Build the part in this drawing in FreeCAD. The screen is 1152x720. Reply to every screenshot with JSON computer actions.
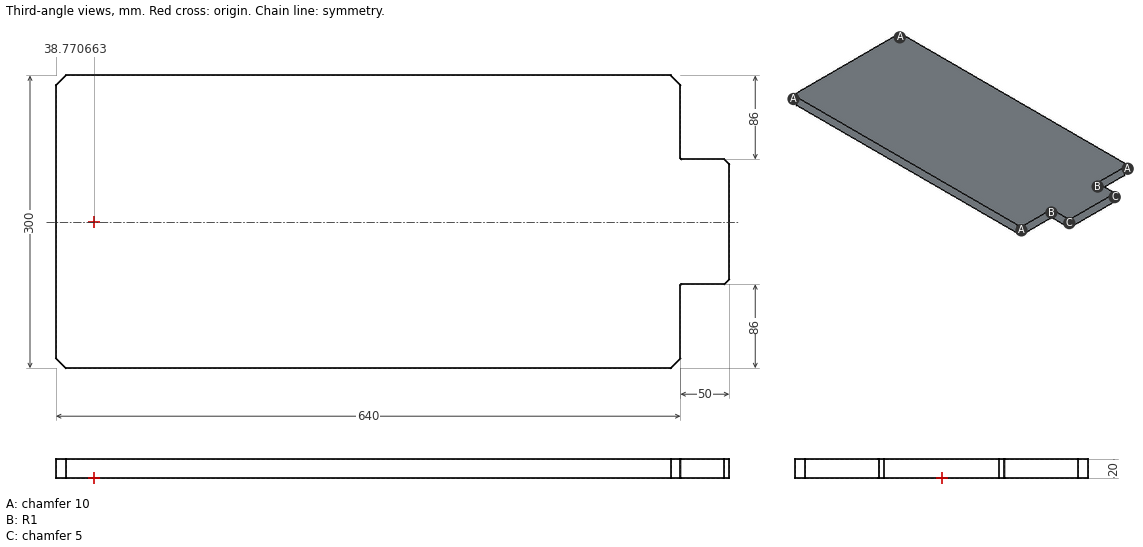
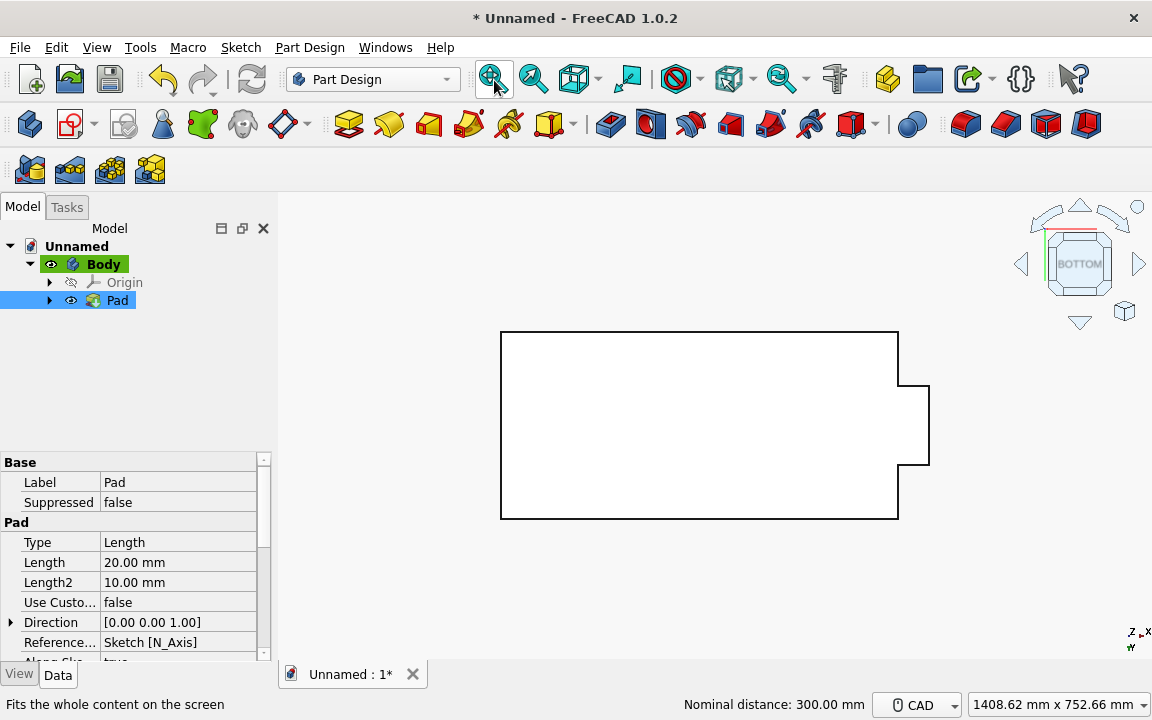
{"action": "scroll", "coordinate": [501, 331], "scroll_direction": "up", "scroll_amount": 6}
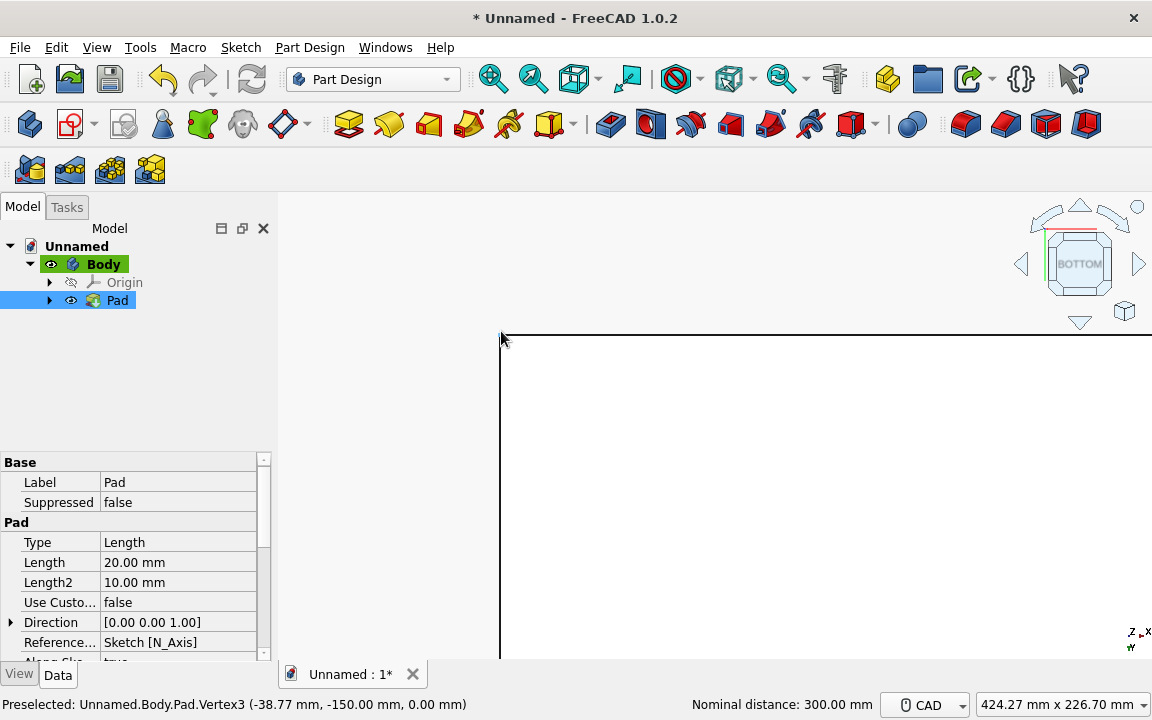
{"action": "left_click", "coordinate": [494, 80]}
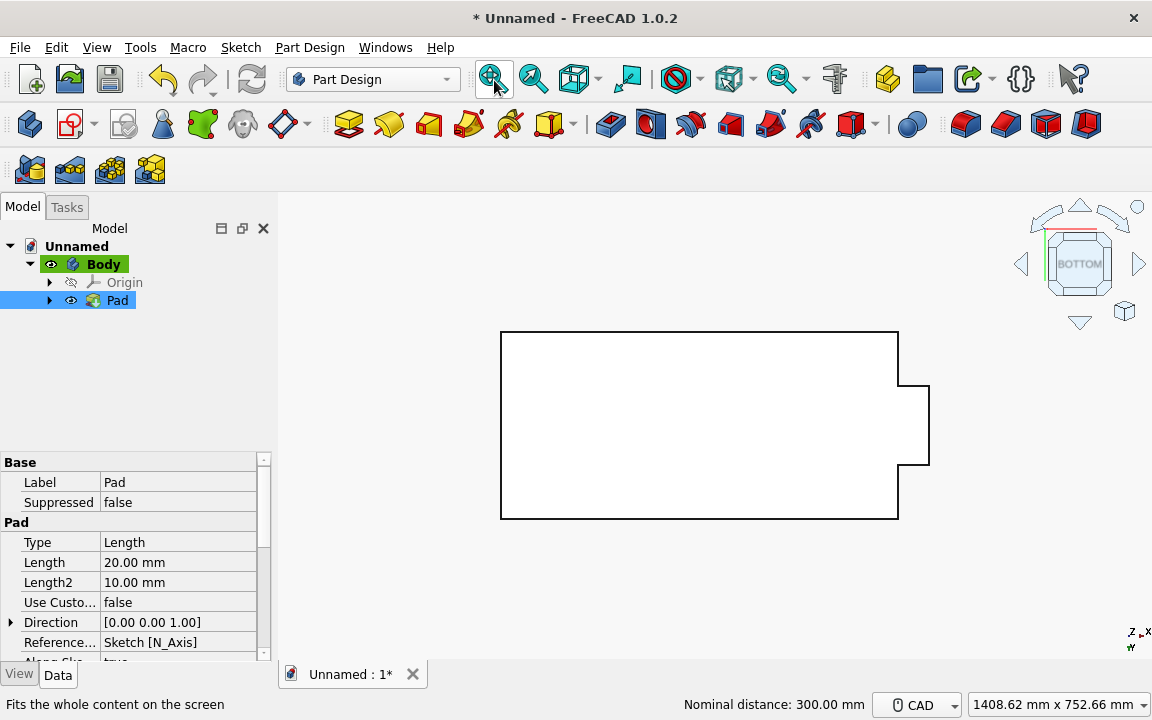
{"action": "key", "text": "4"}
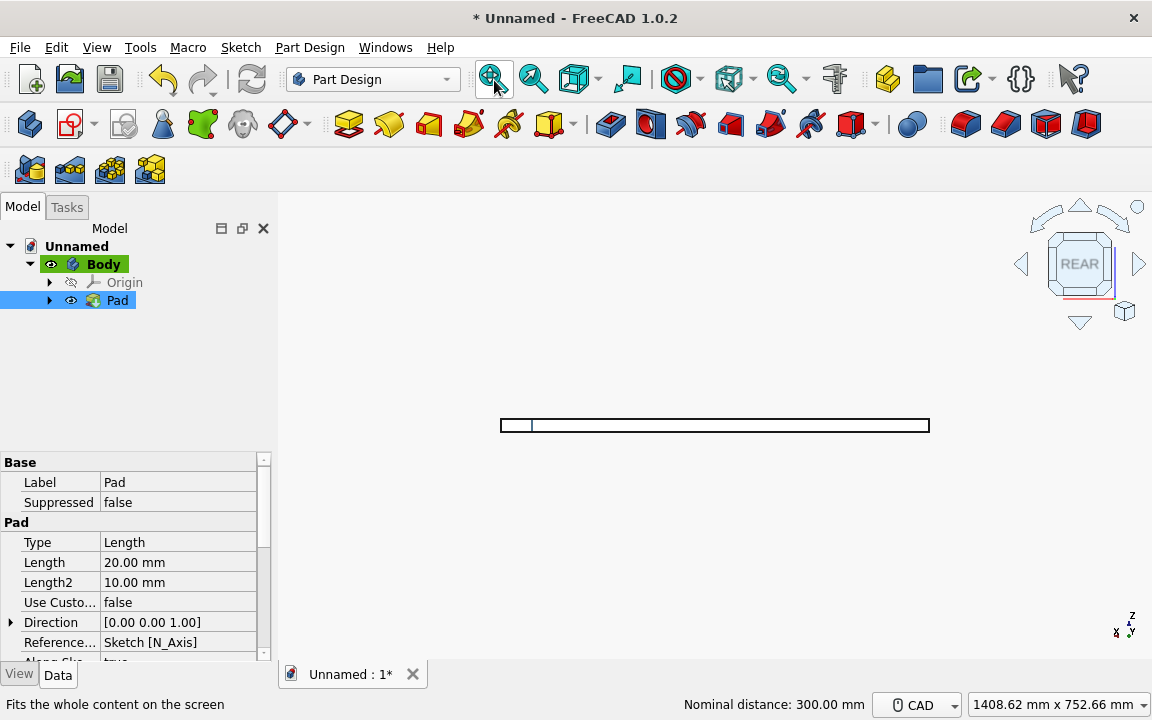
{"action": "scroll", "coordinate": [929, 424], "scroll_direction": "up", "scroll_amount": 6}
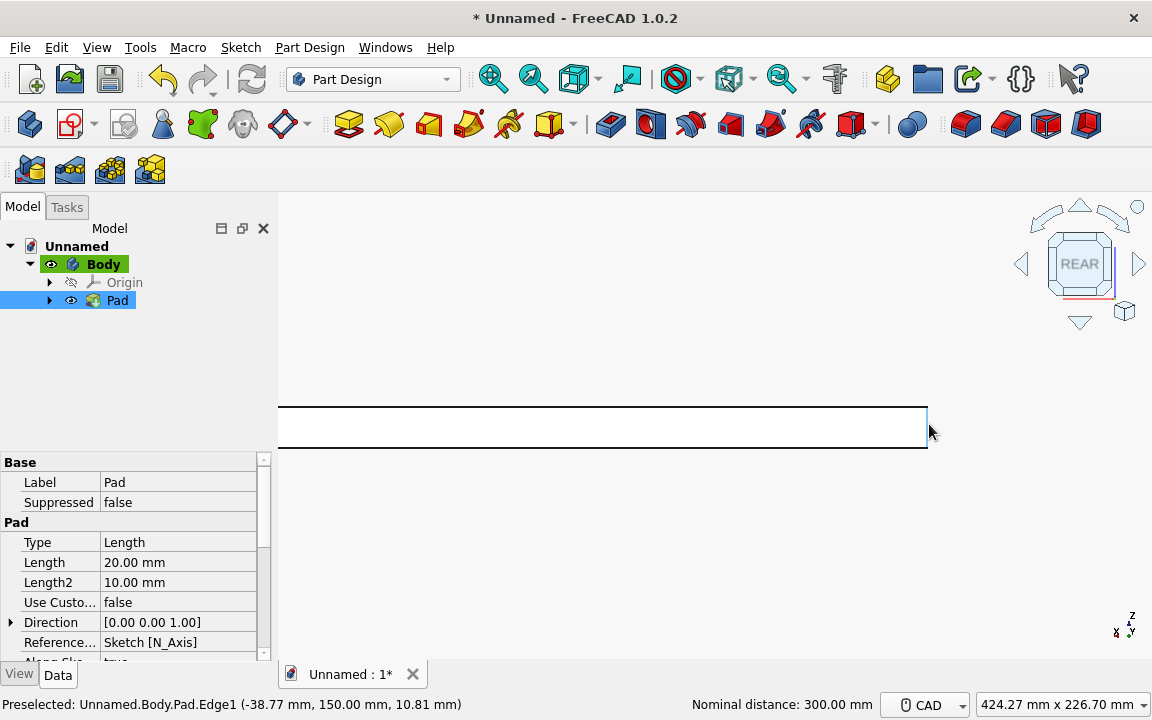
{"action": "left_click", "coordinate": [927, 427], "text": "ctrl"}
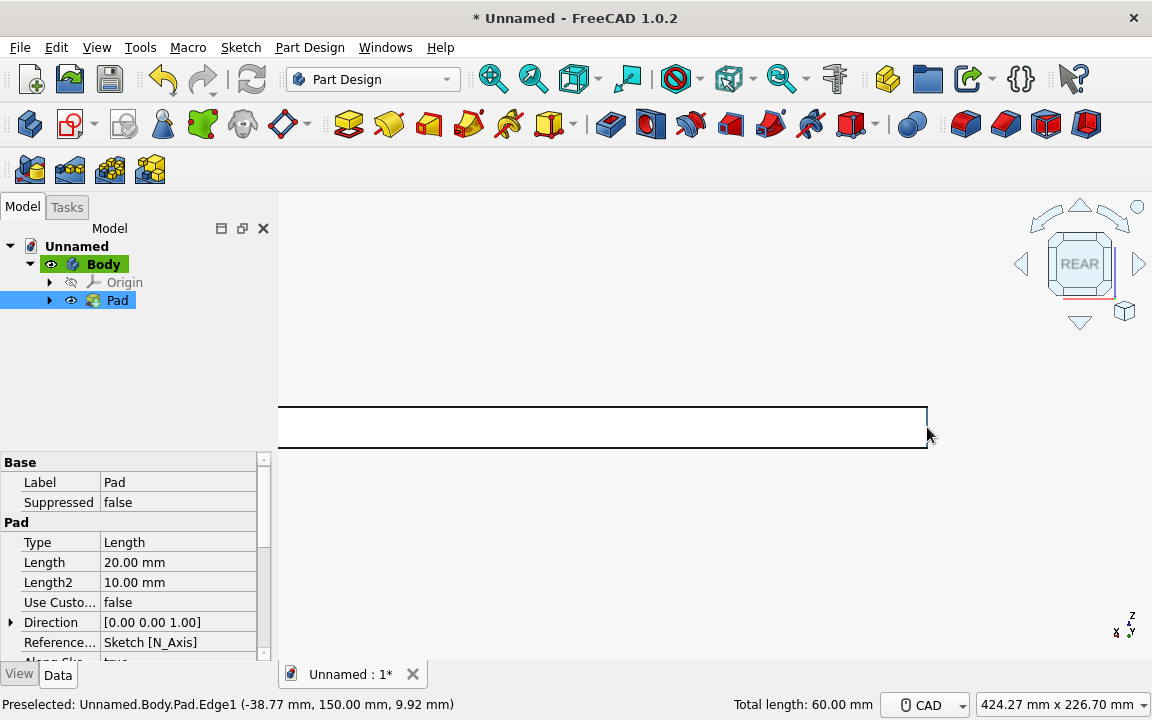
{"action": "left_click", "coordinate": [494, 80]}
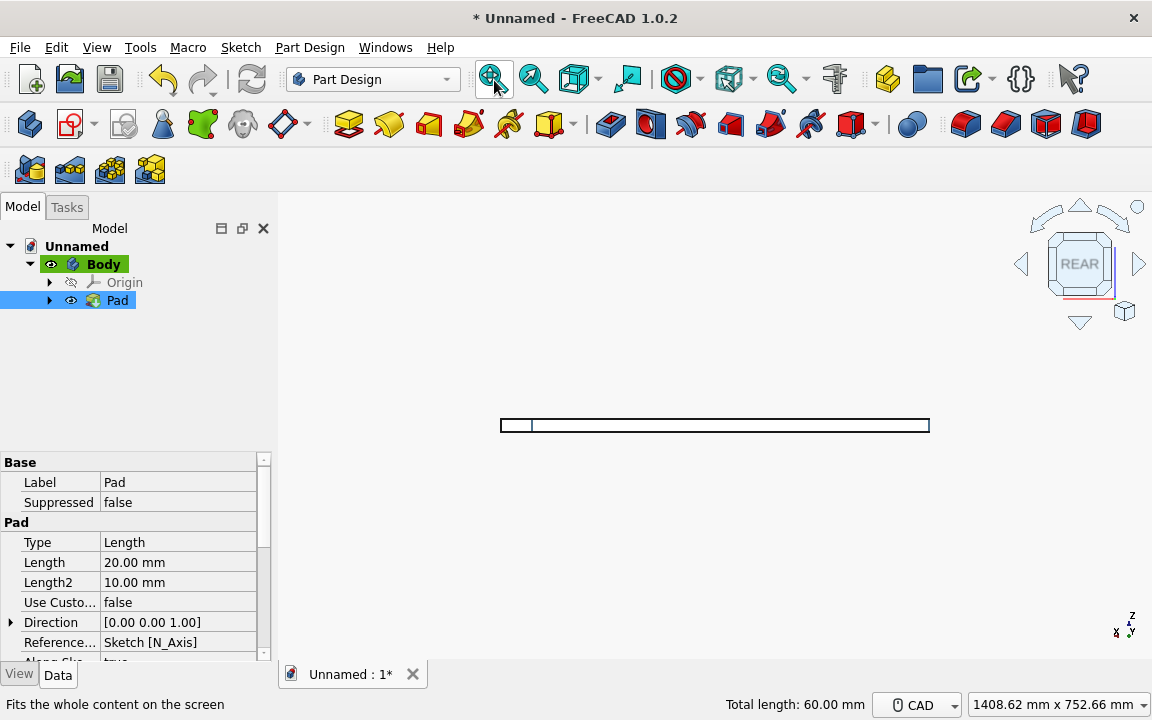
{"action": "key", "text": "6"}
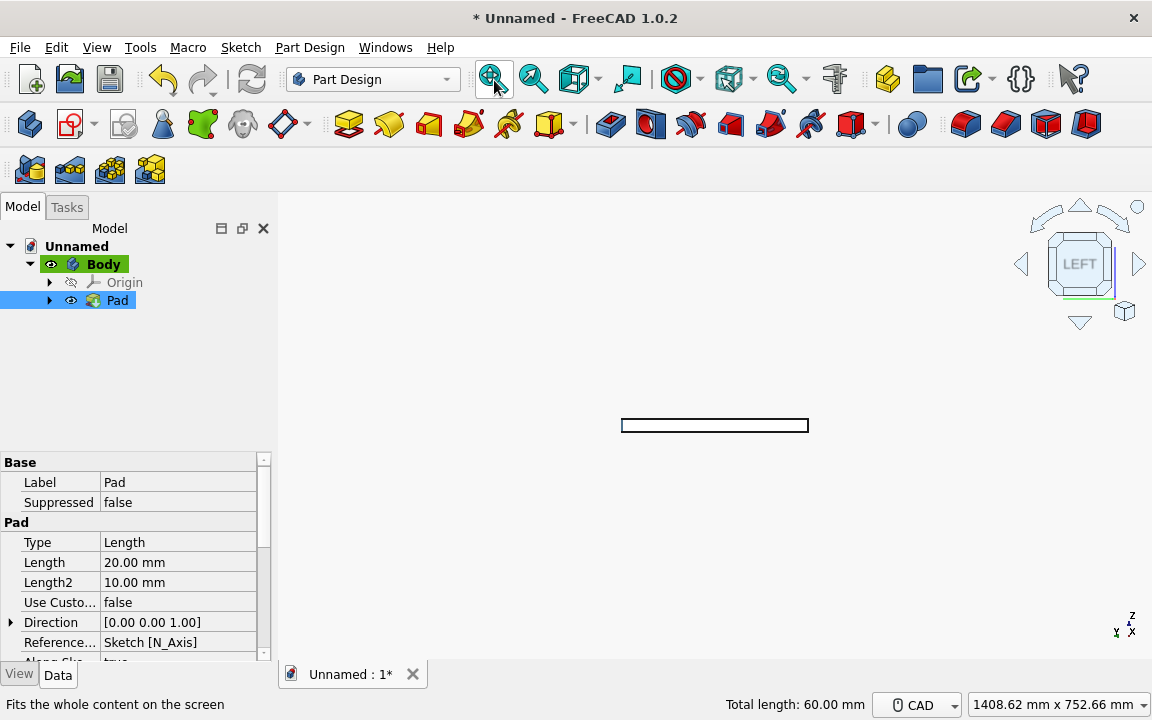
{"action": "left_click", "coordinate": [494, 80]}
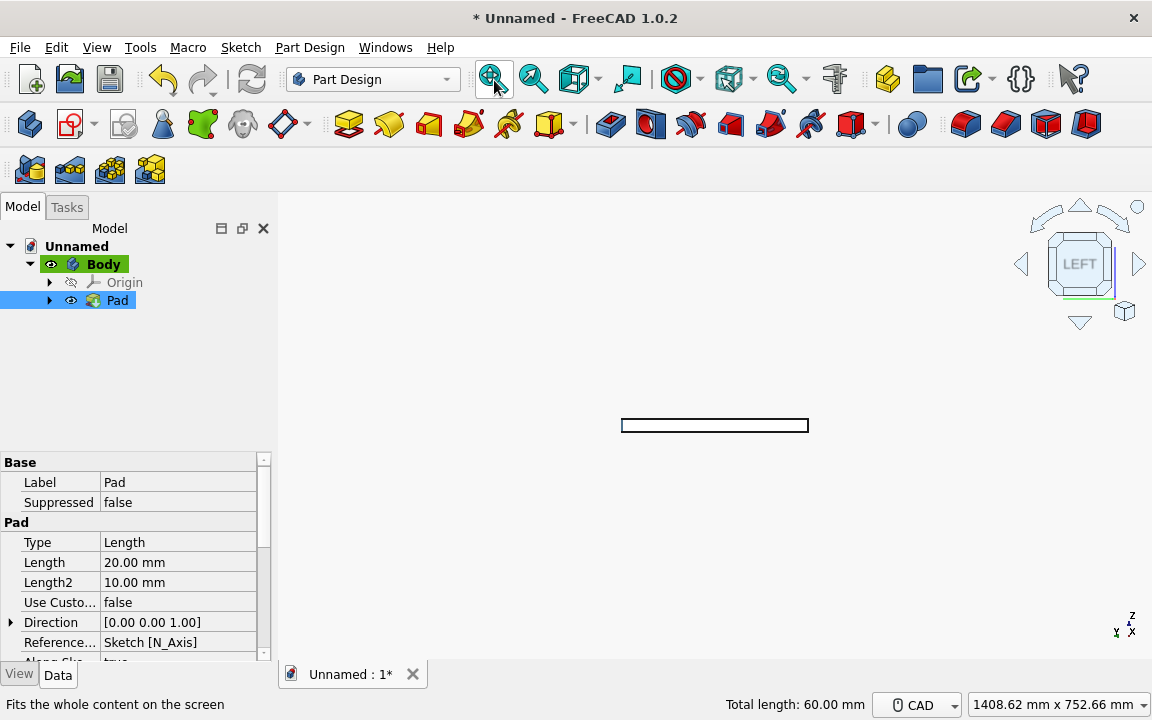
{"action": "scroll", "coordinate": [808, 424], "scroll_direction": "up", "scroll_amount": 6}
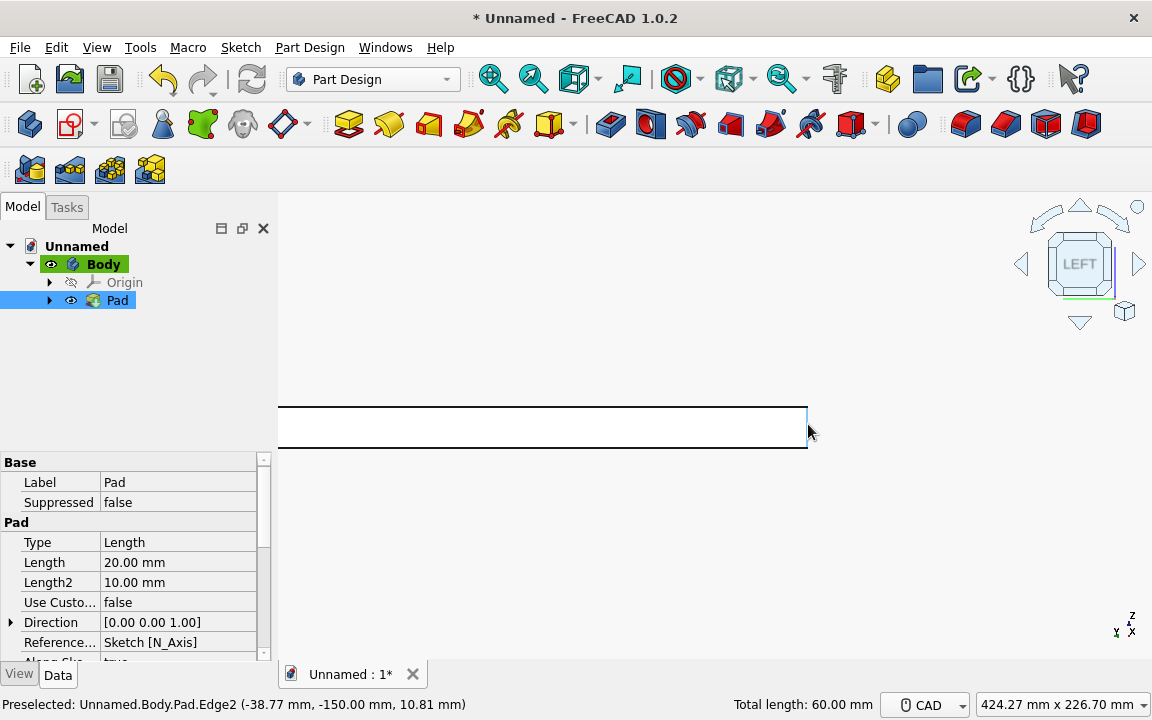
{"action": "left_click", "coordinate": [807, 427], "text": "ctrl"}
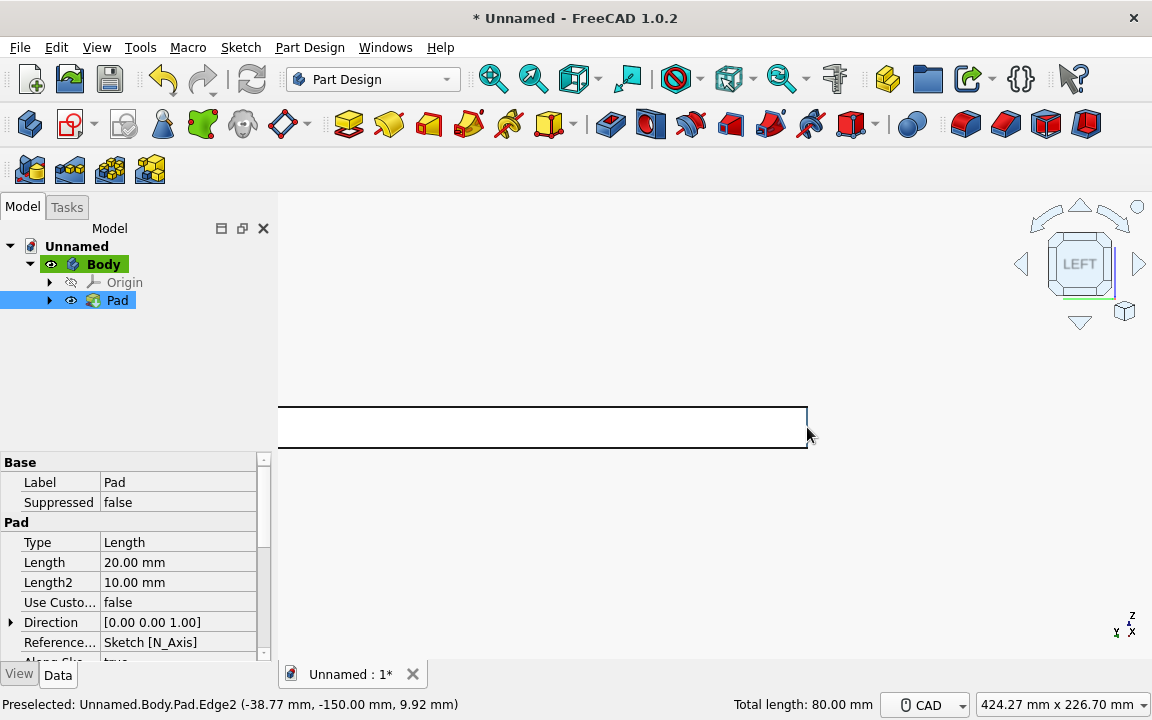
{"action": "left_click", "coordinate": [1006, 124]}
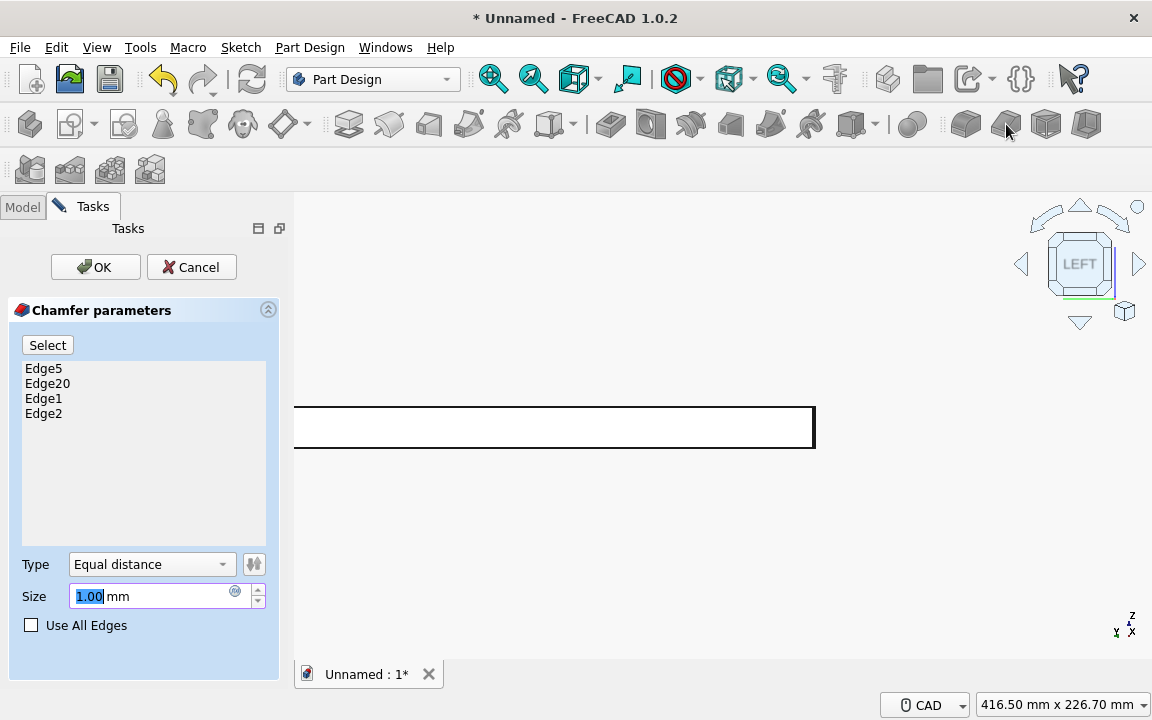
{"action": "type", "text": "10"}
{"action": "key", "text": "Tab"}